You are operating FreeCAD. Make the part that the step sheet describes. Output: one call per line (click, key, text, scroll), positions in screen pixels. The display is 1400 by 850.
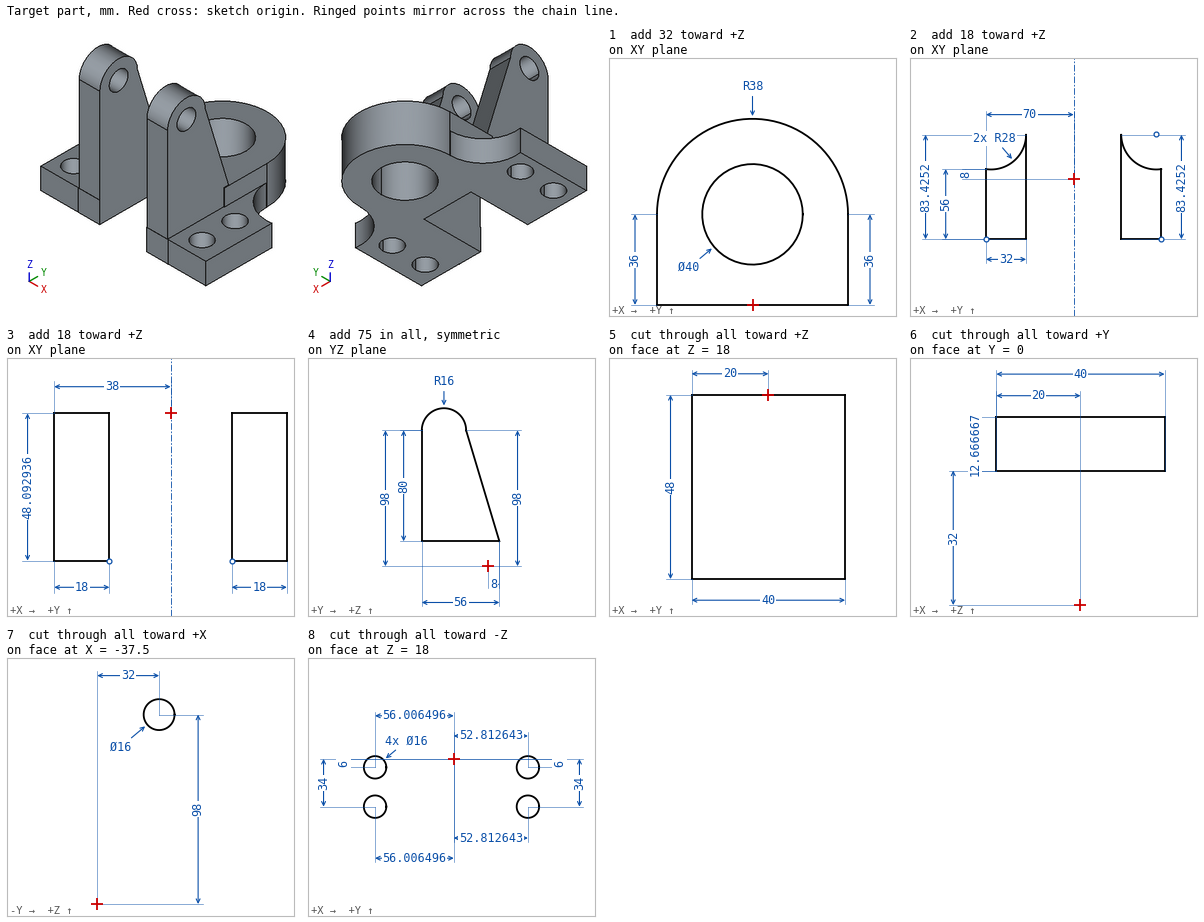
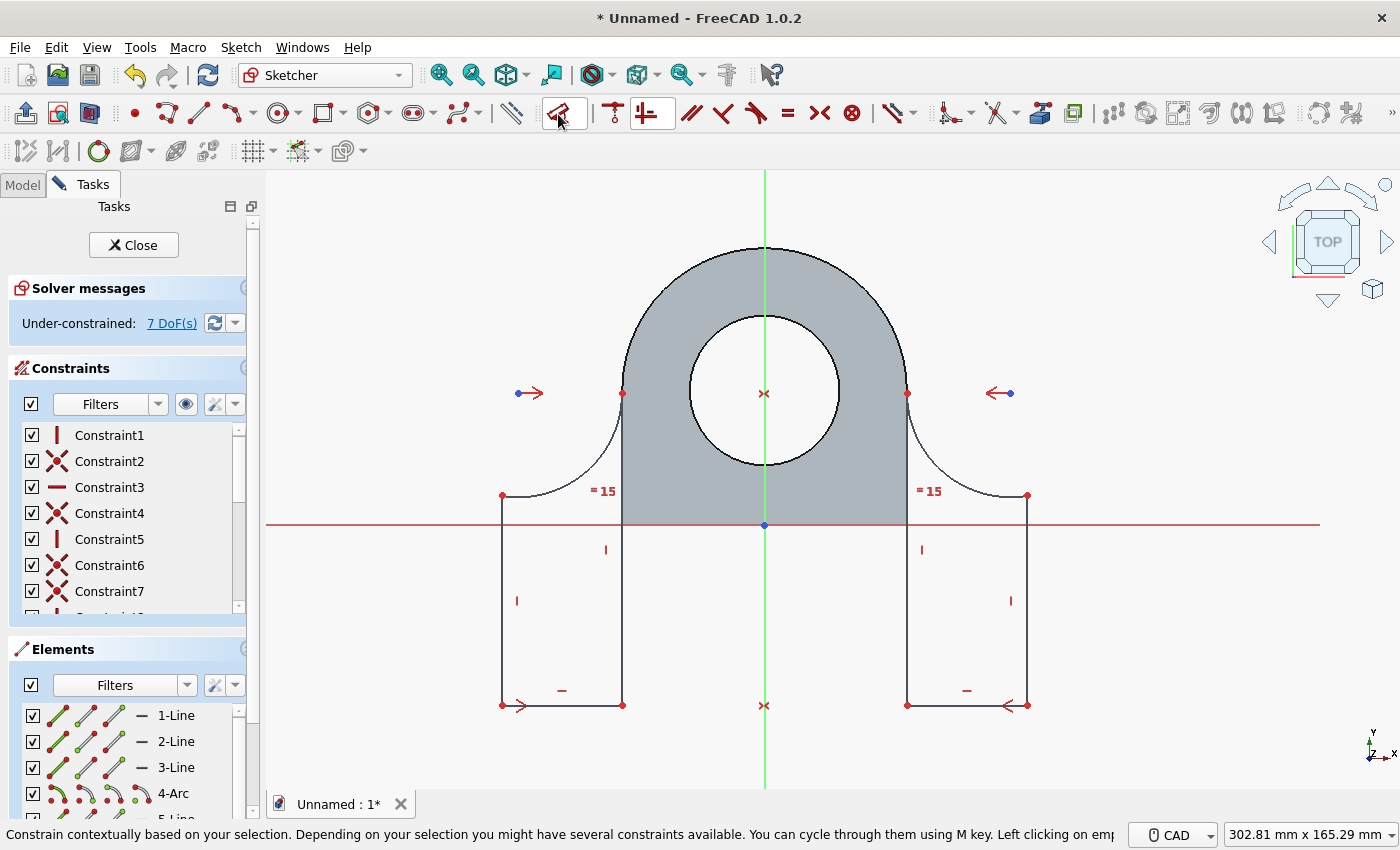
click(555, 491)
click(437, 503)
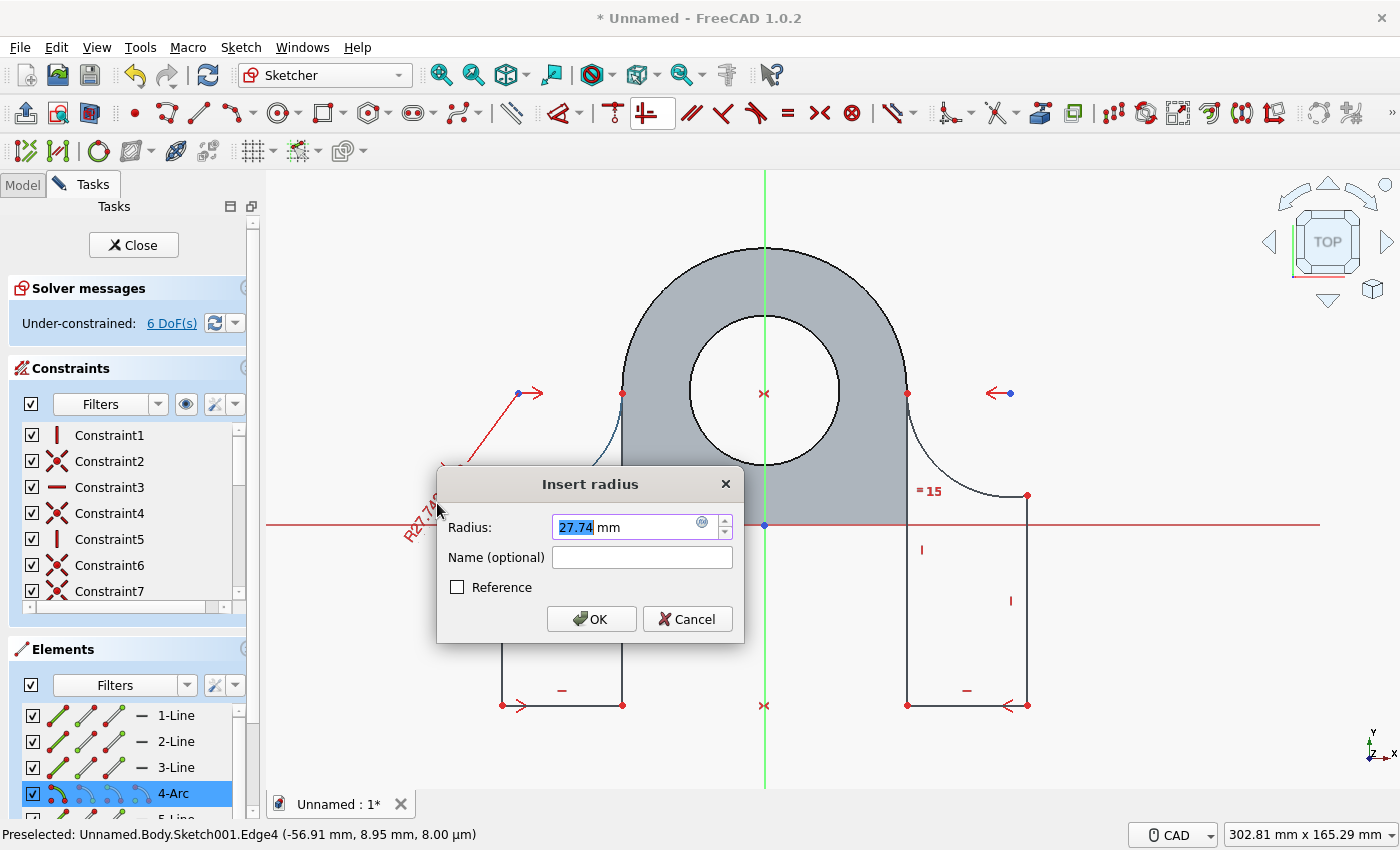
text(28)
key(Return)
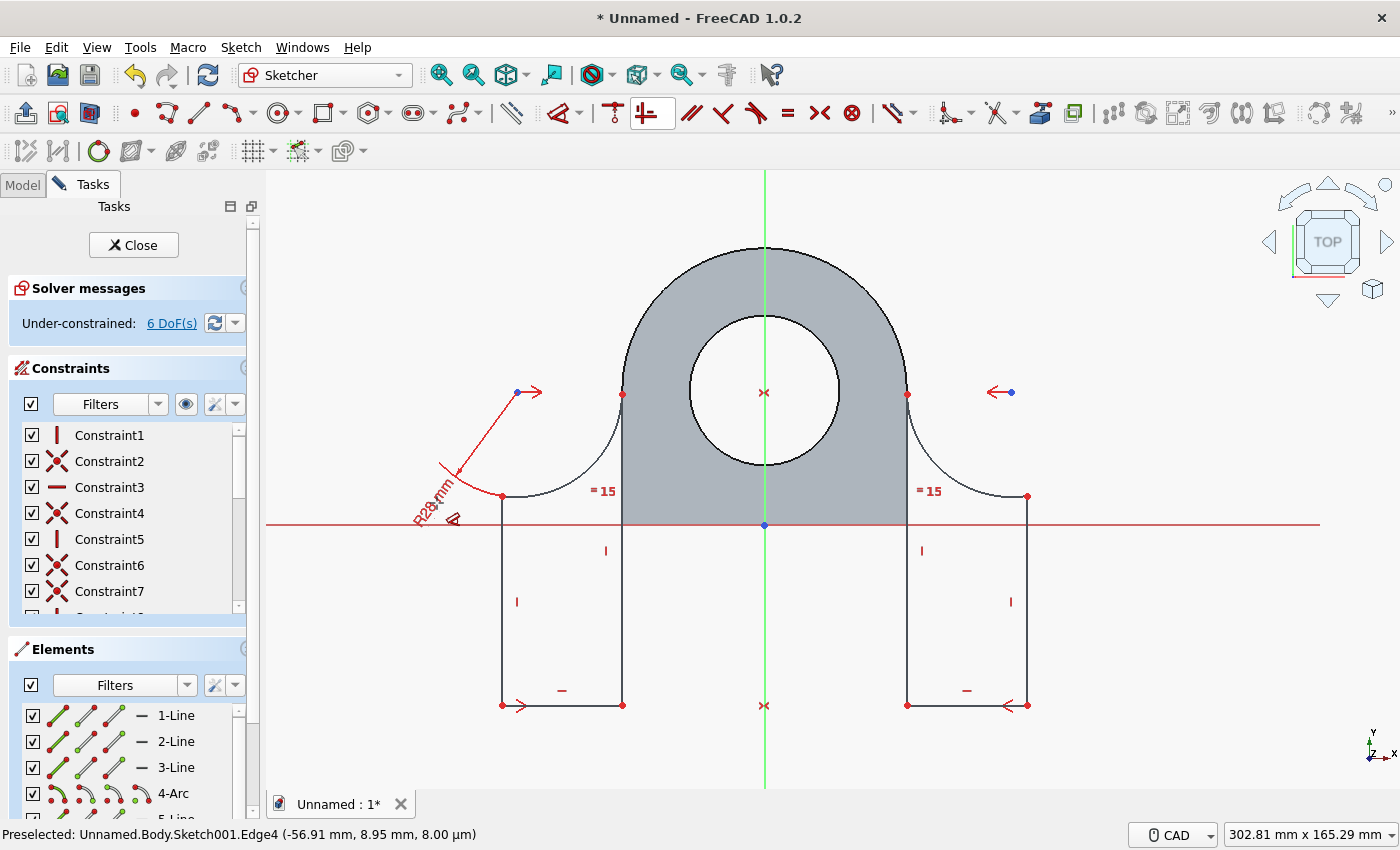
click(502, 559)
click(468, 601)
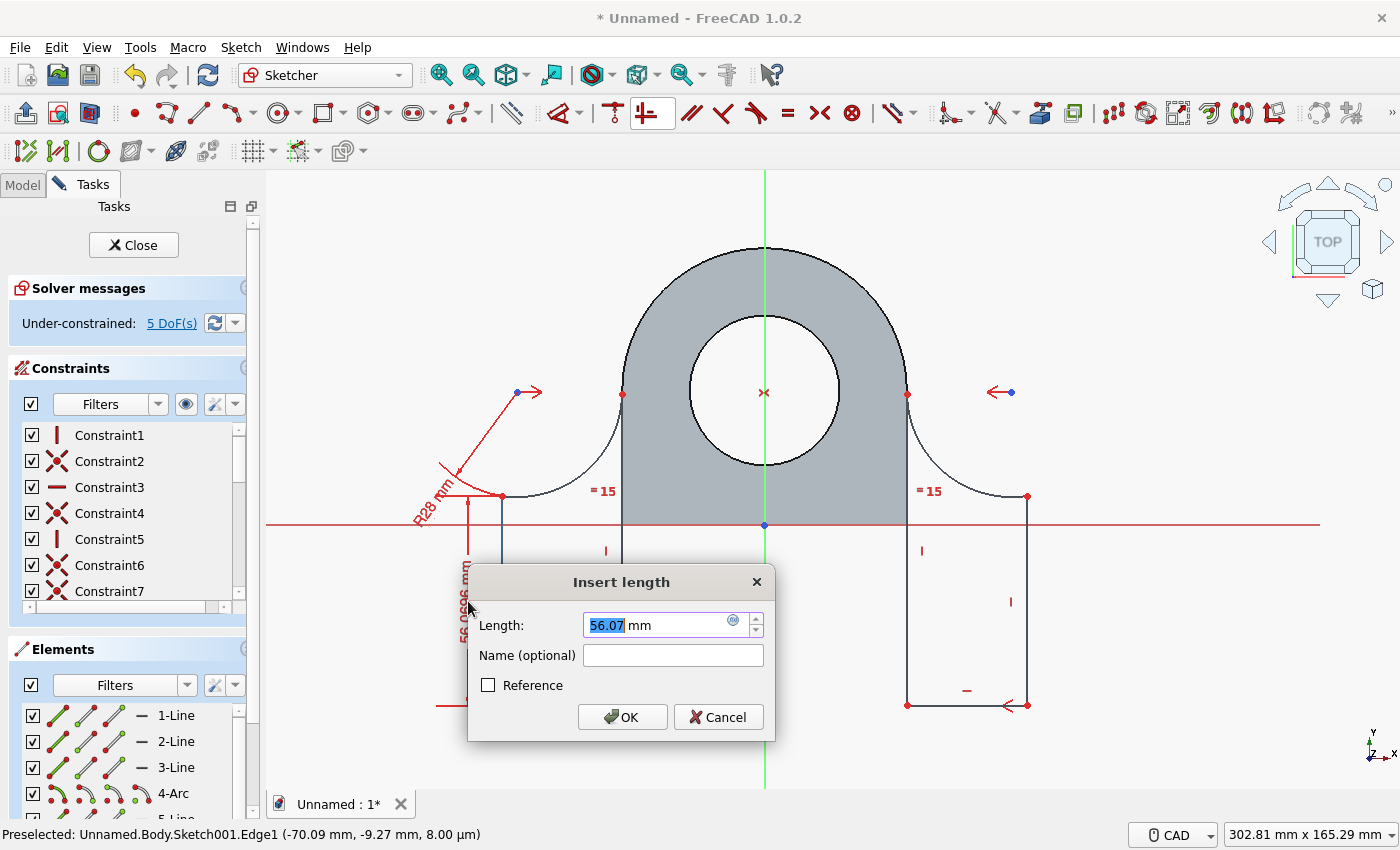
text(56)
key(Return)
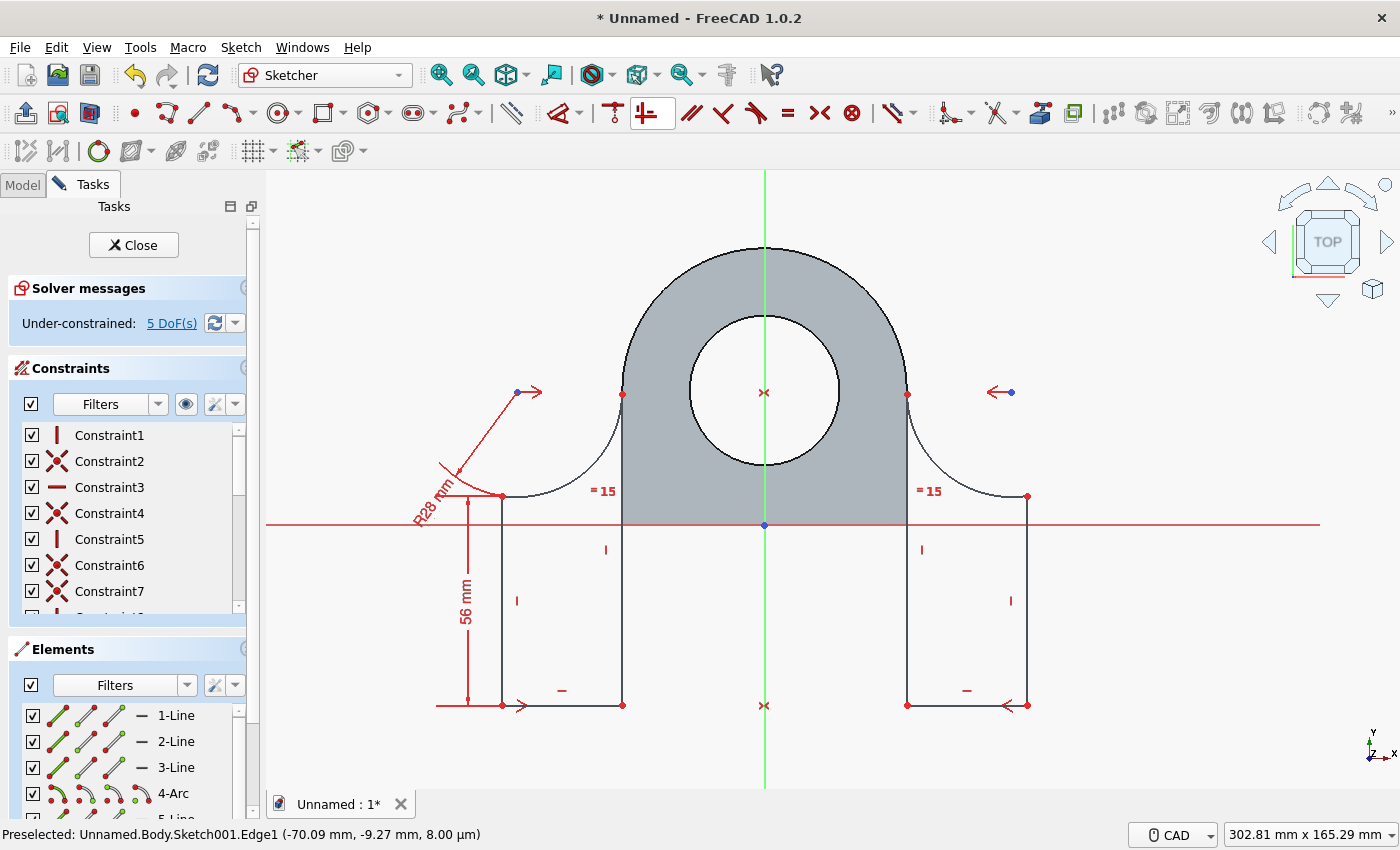
click(538, 706)
click(562, 740)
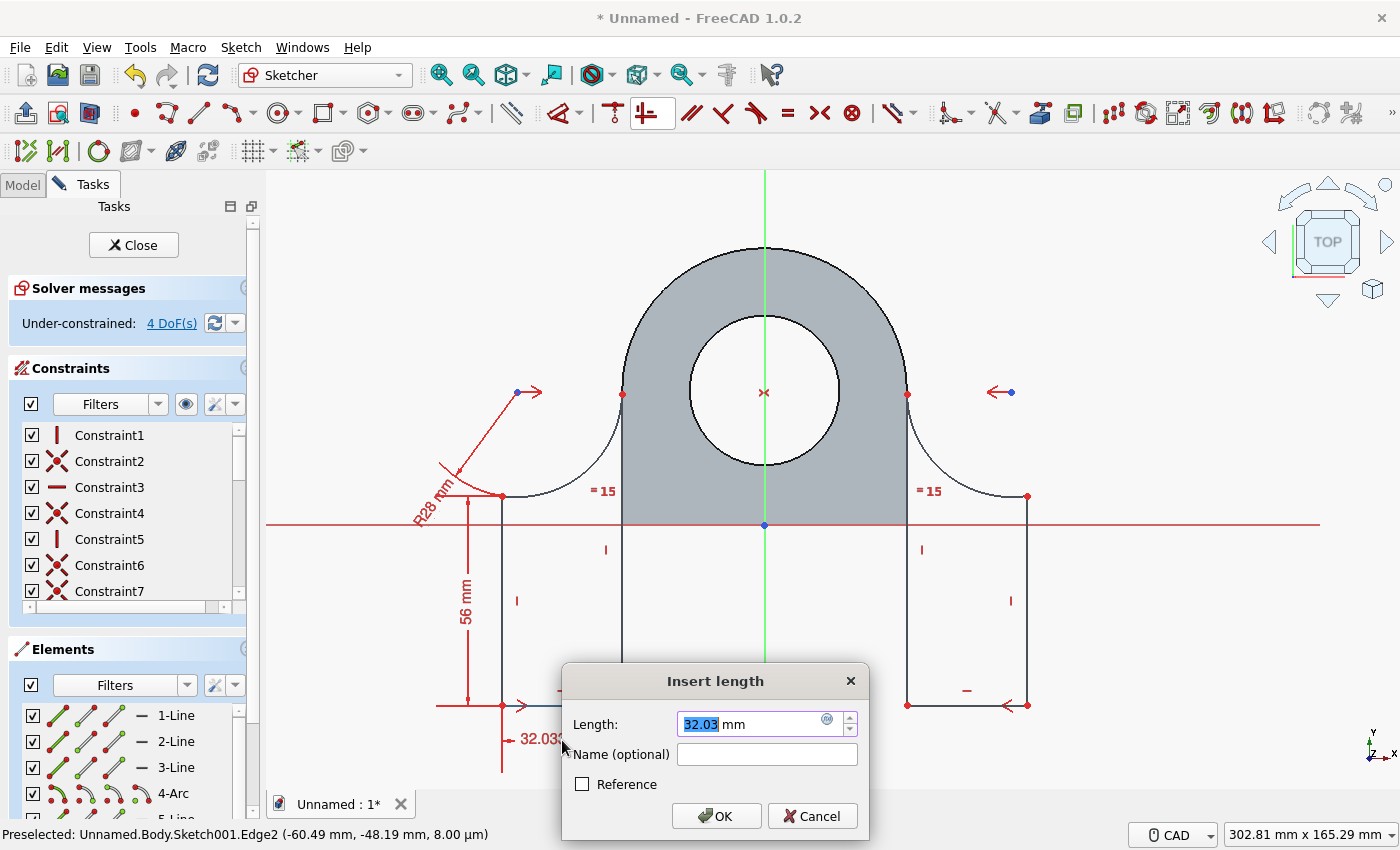
text(32)
key(Return)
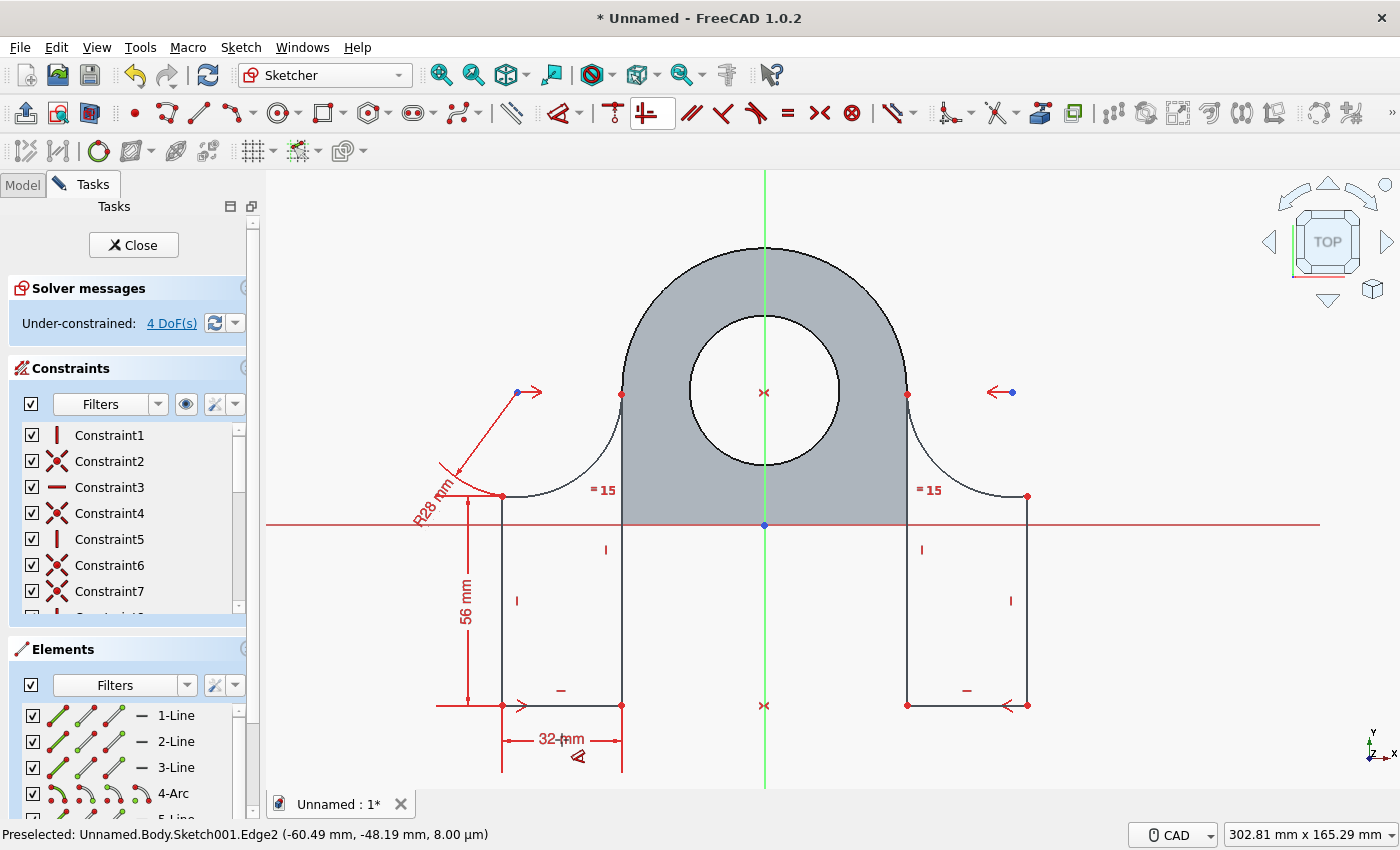
scroll(502, 496, up, 2)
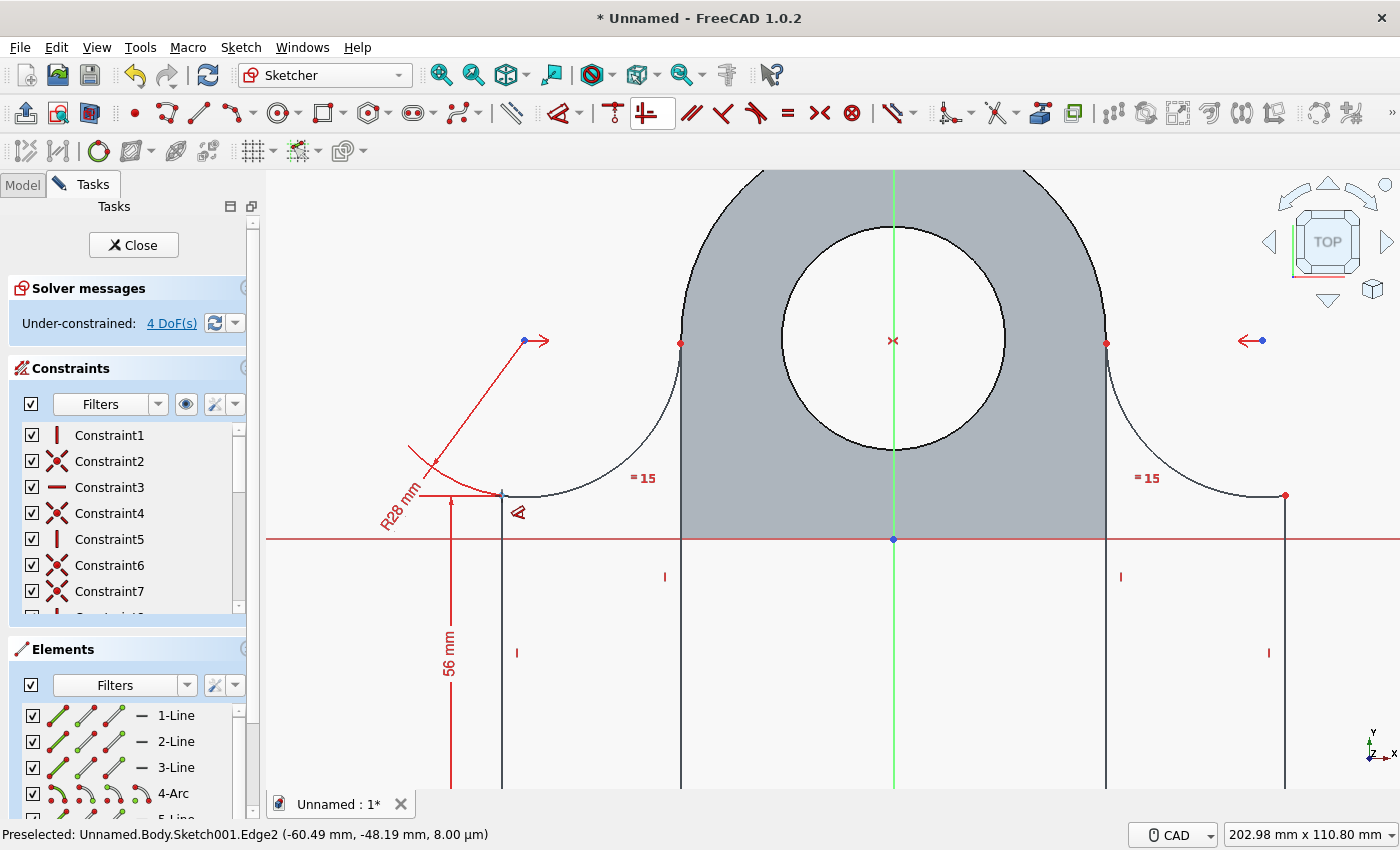
click(502, 496)
click(928, 518)